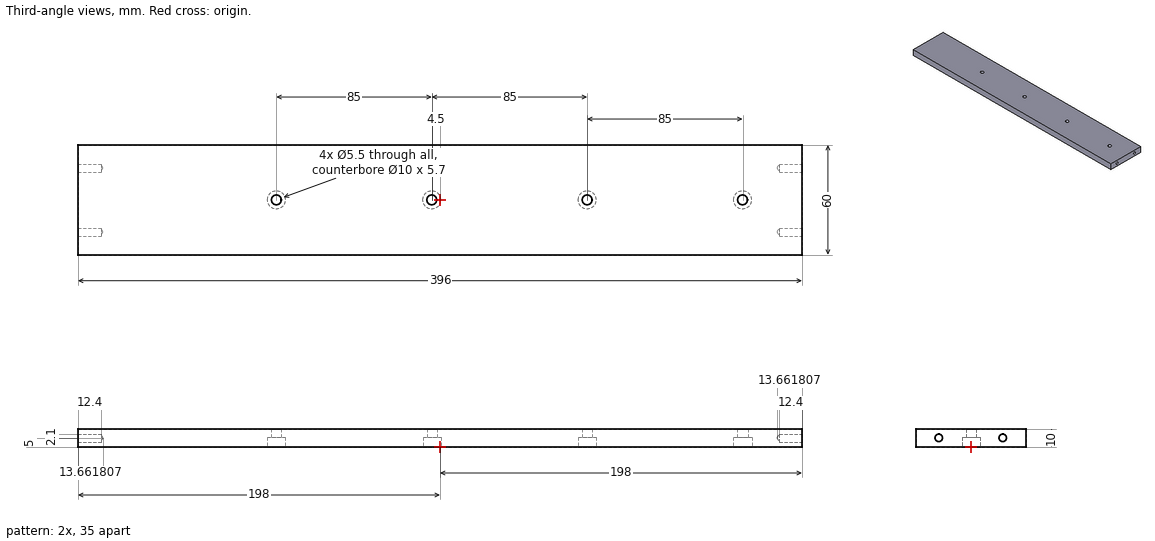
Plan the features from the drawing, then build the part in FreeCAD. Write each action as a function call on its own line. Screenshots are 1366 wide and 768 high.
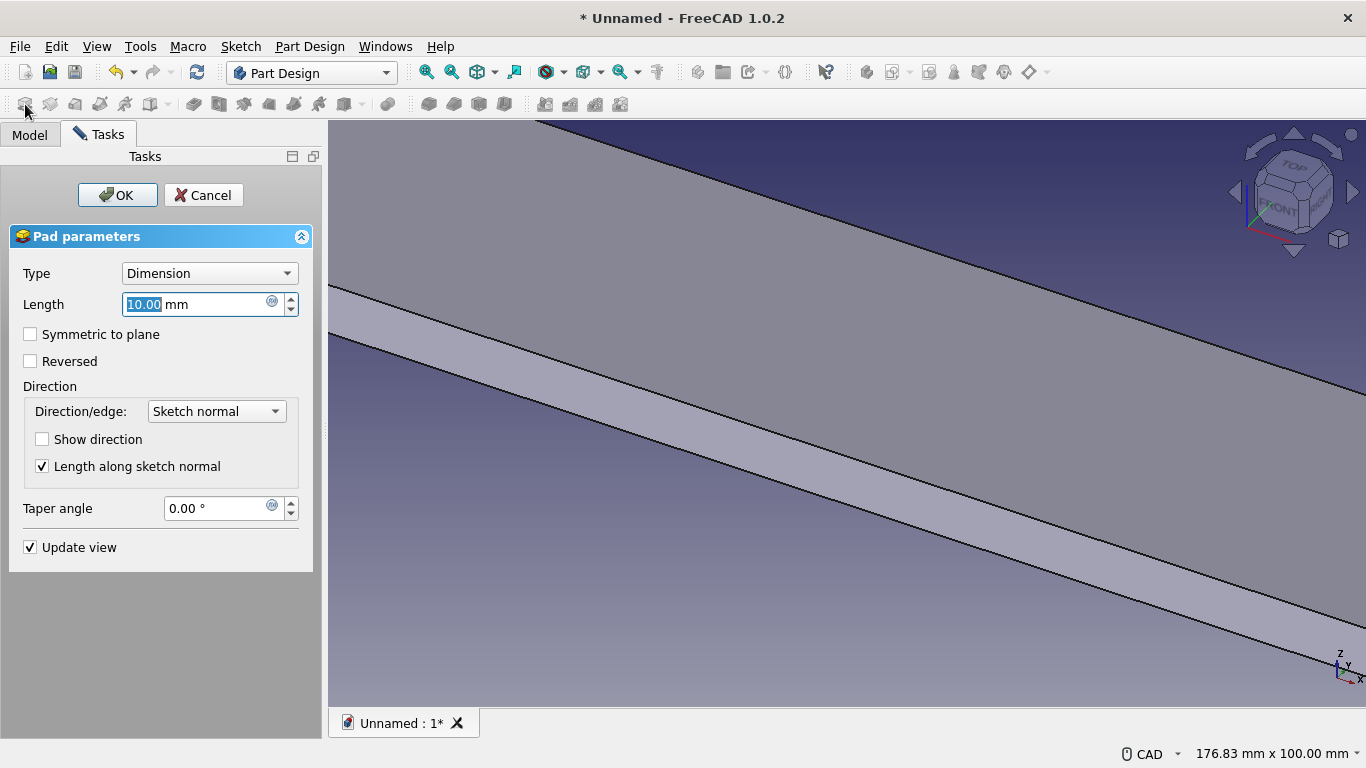
text(10)
key(Tab)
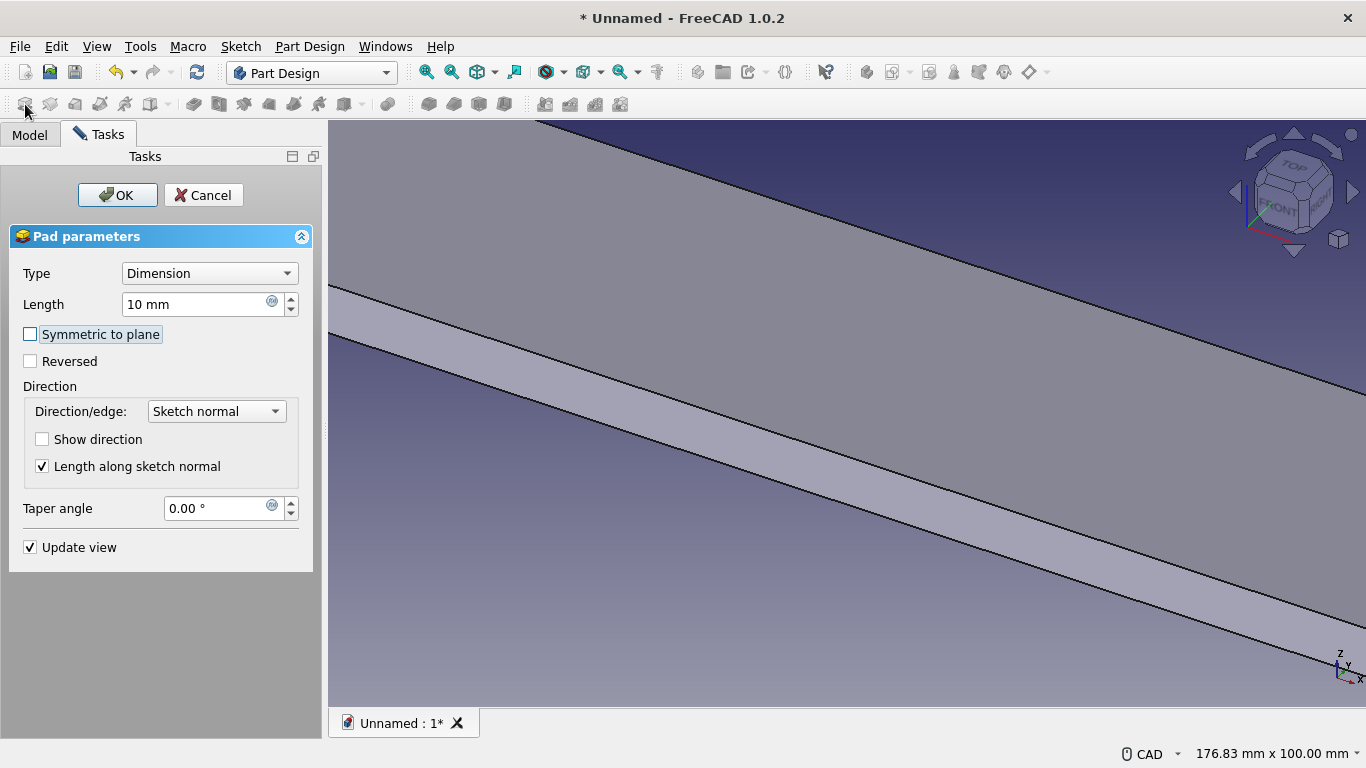
click(118, 195)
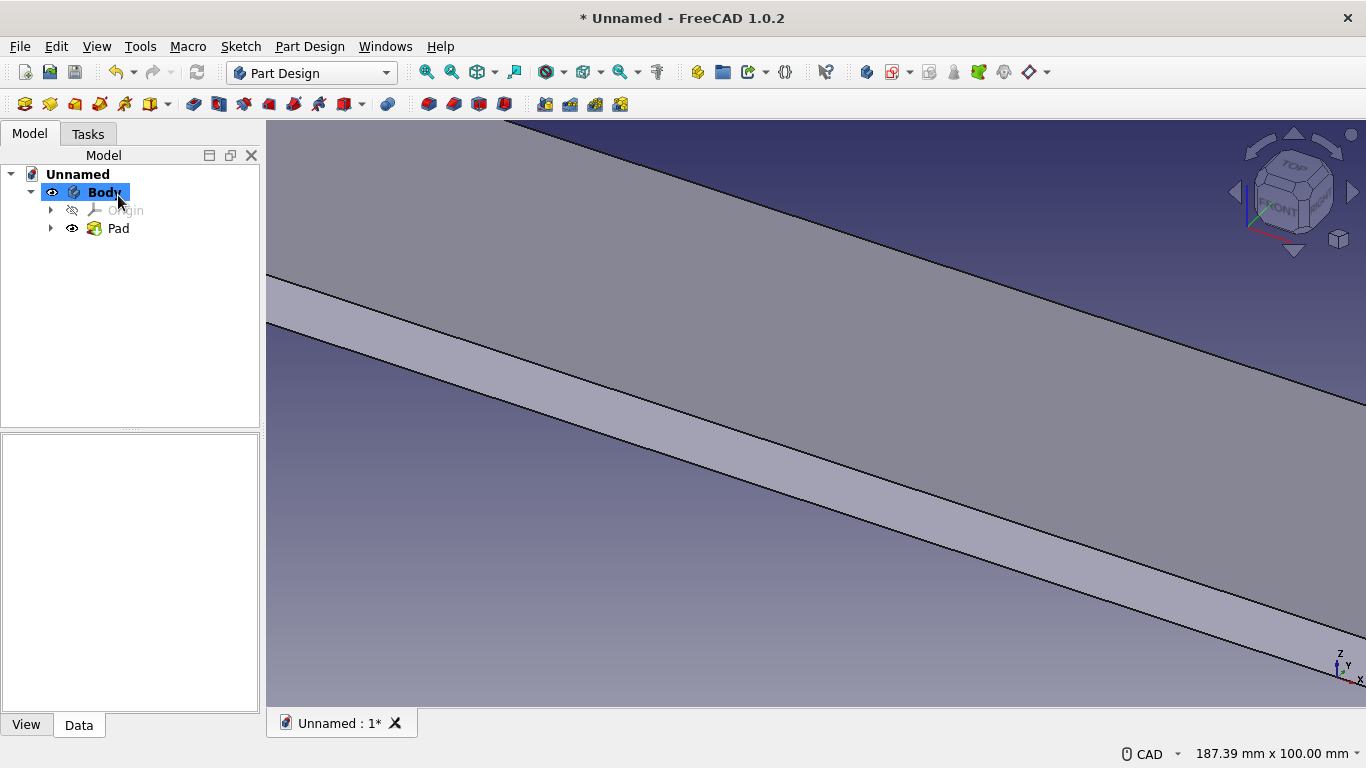
click(427, 72)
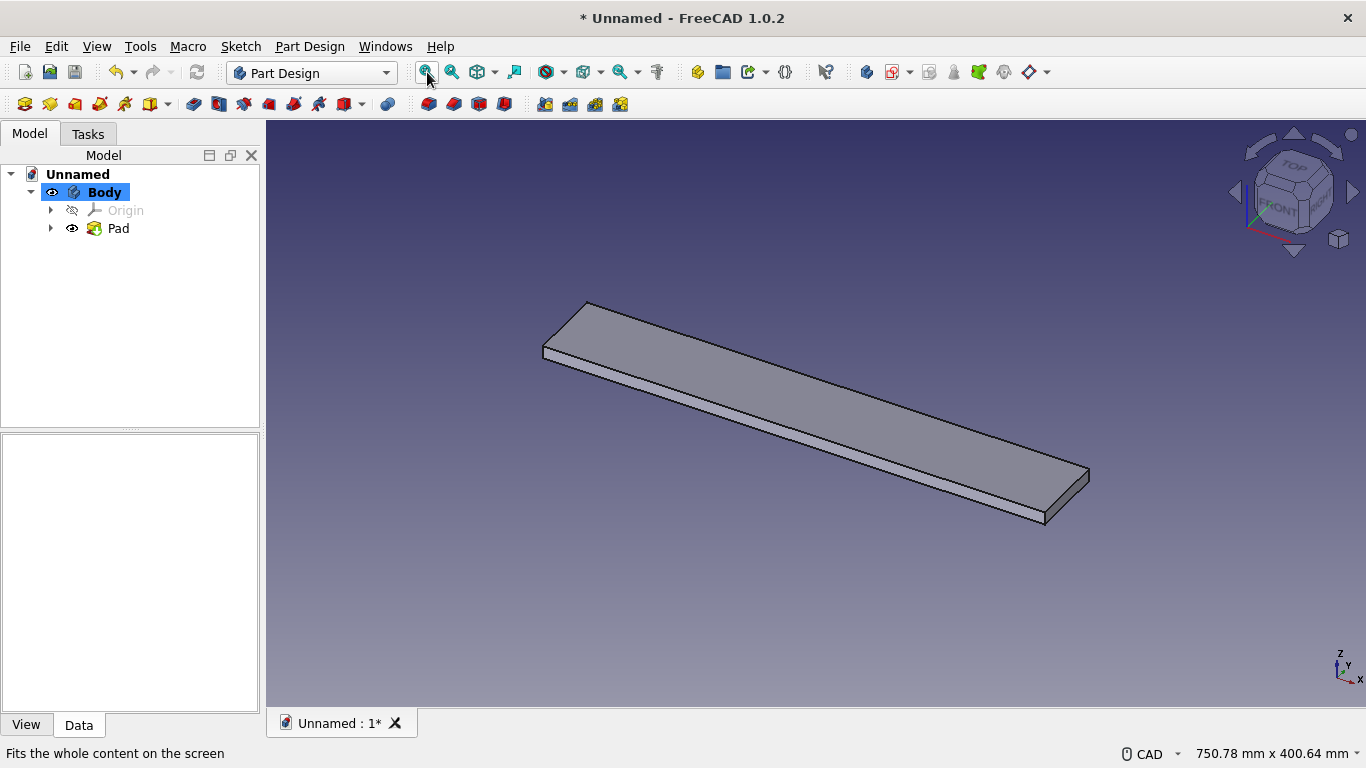
click(892, 72)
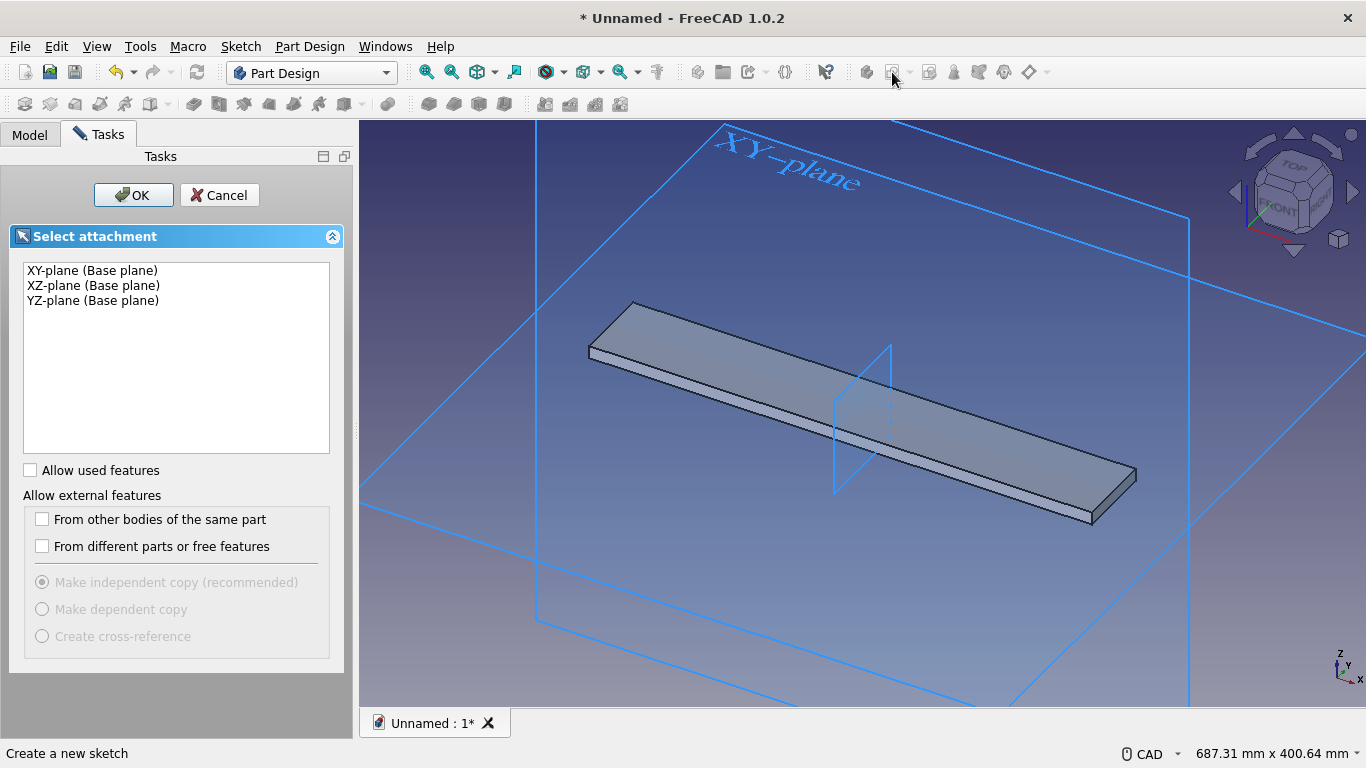
click(84, 270)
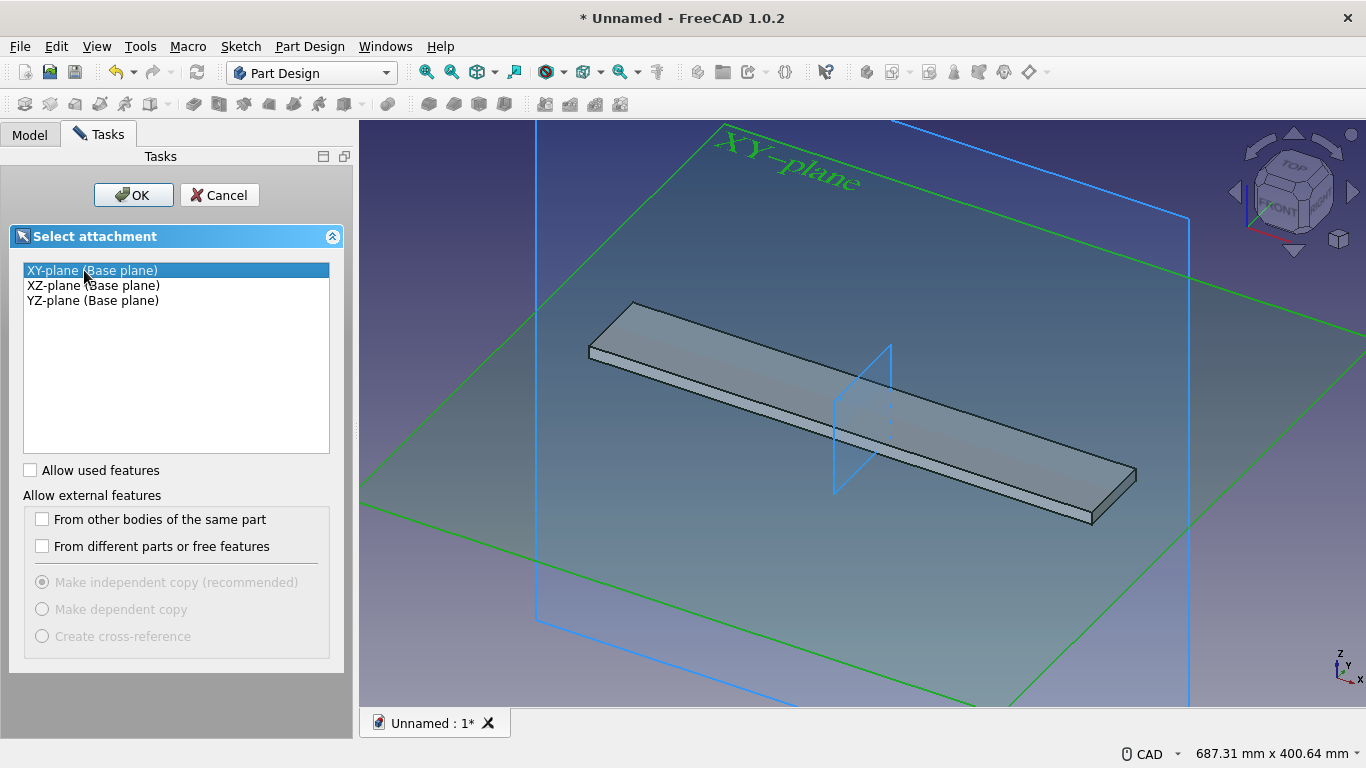
click(134, 195)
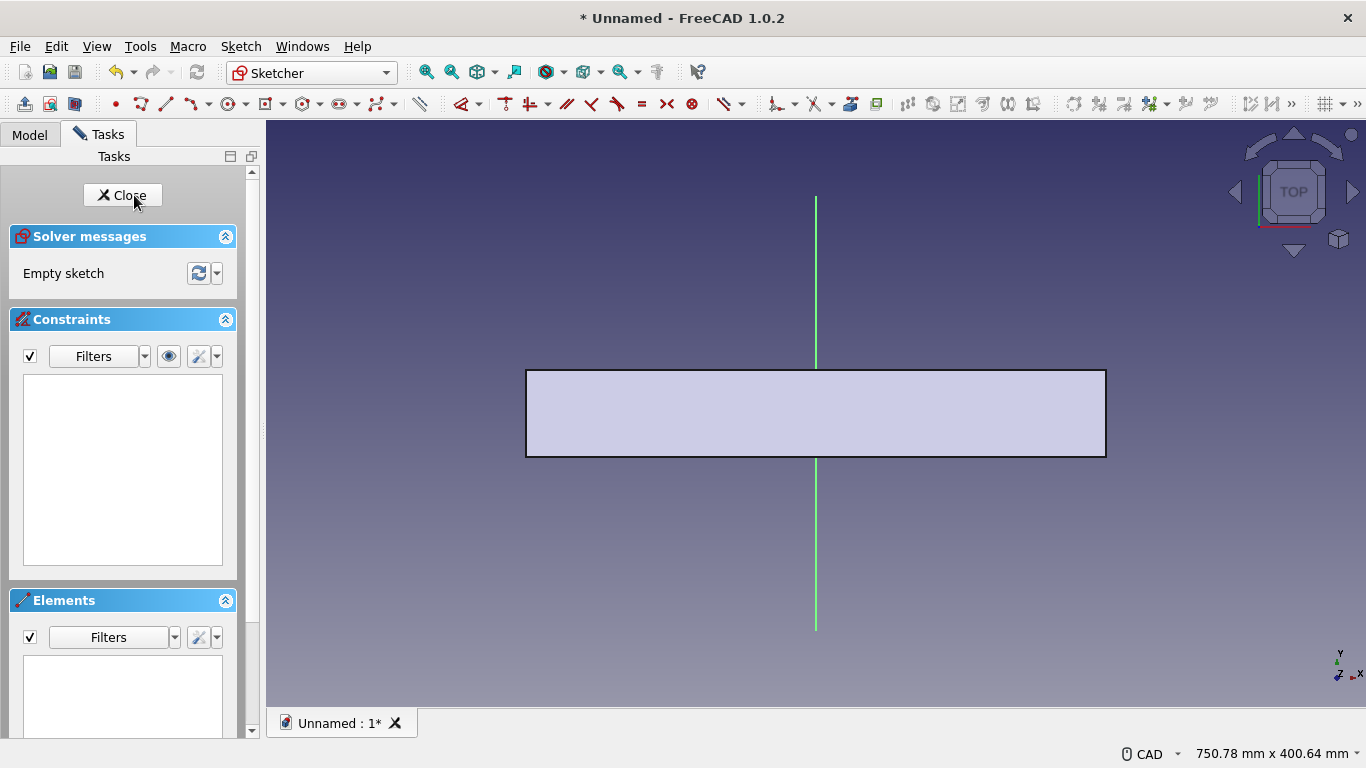
click(75, 104)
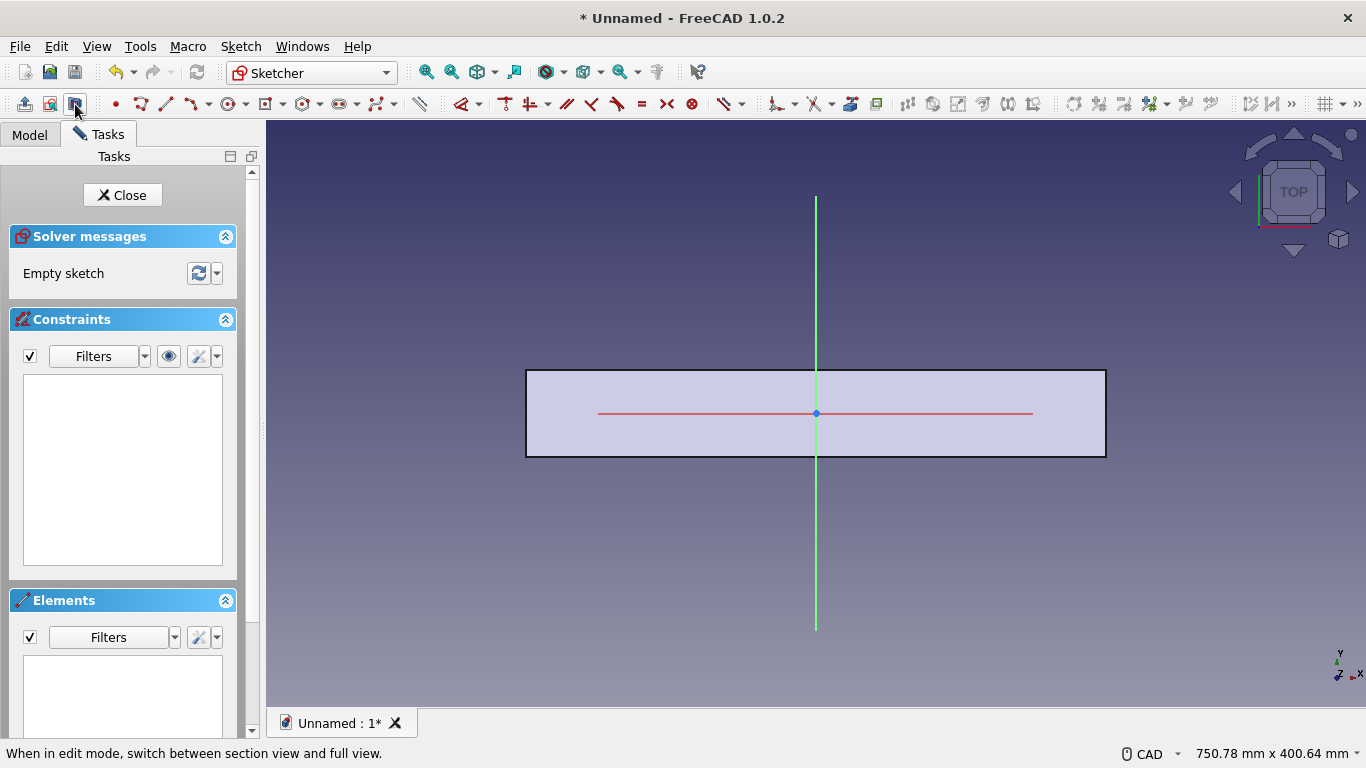
scroll(1023, 414, up, 3)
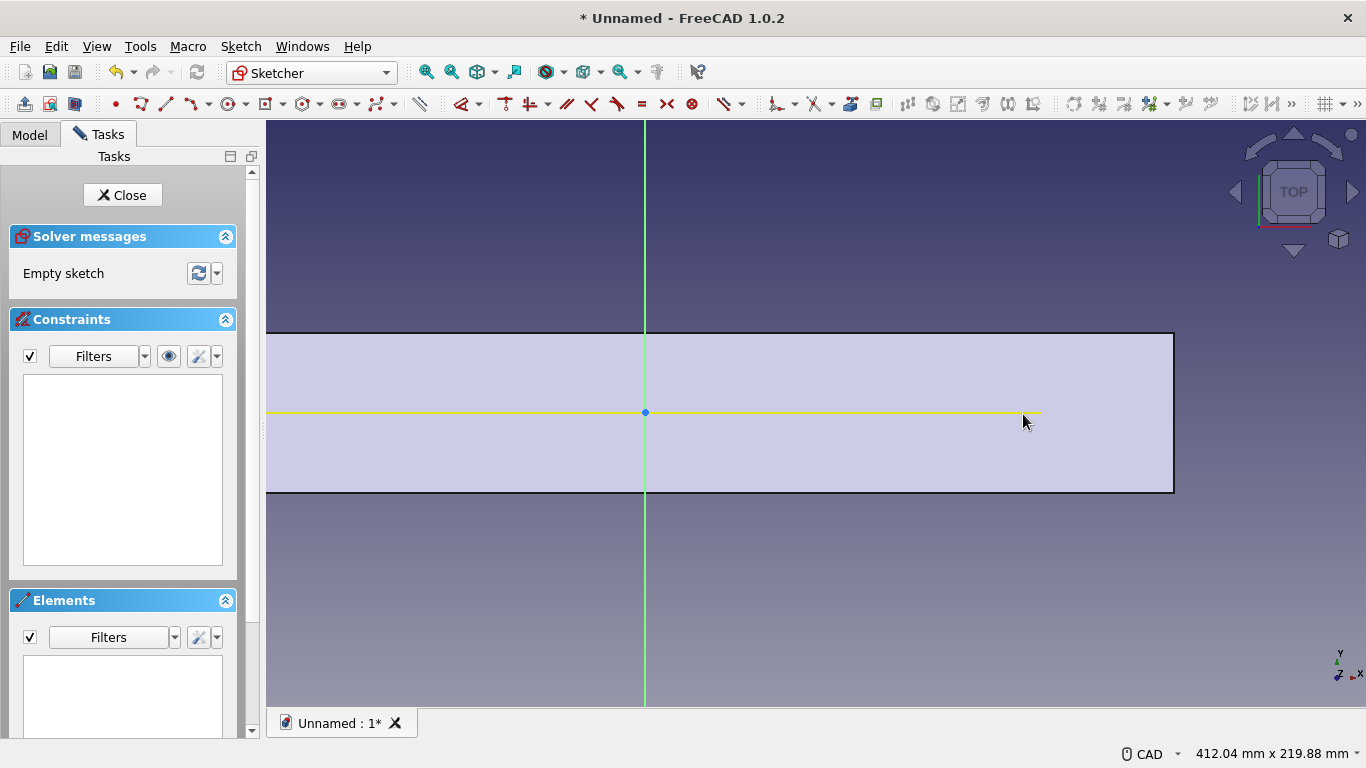
click(228, 104)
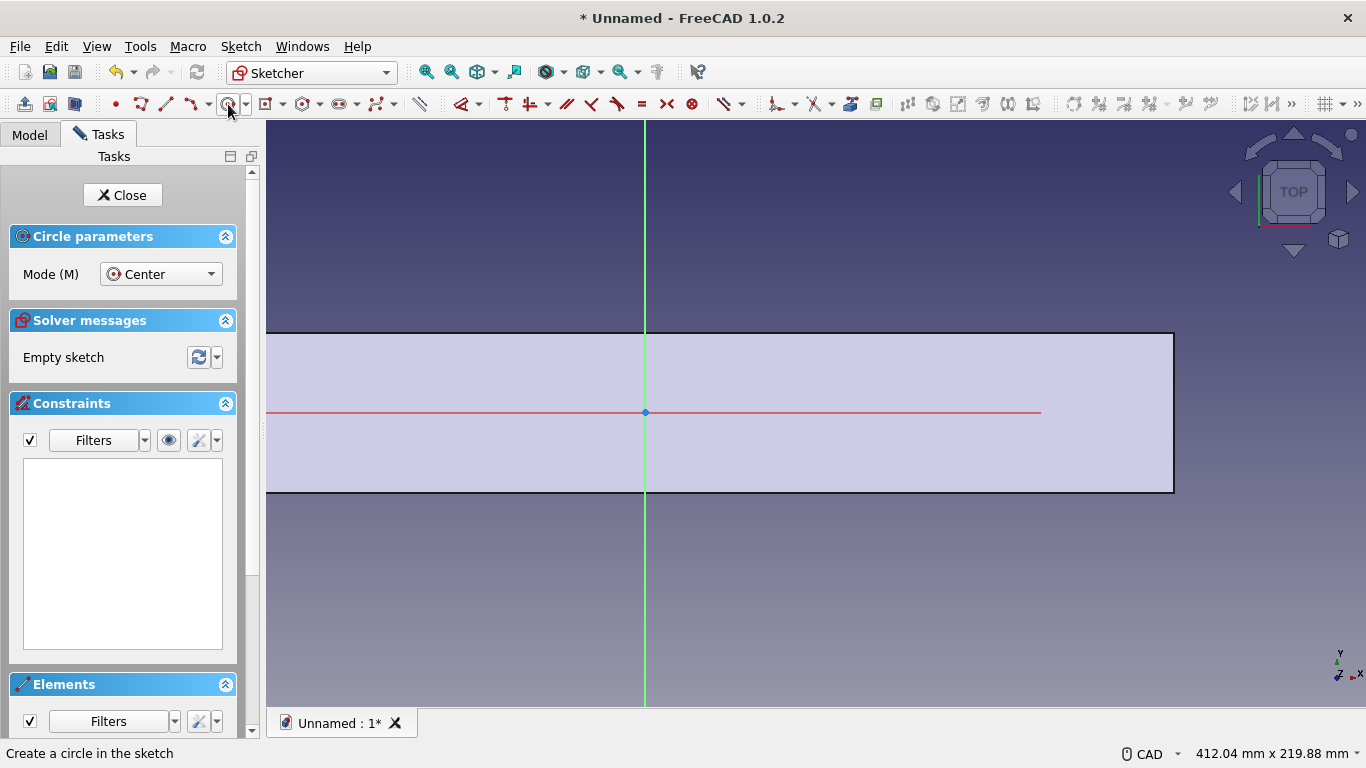
scroll(406, 413, up, 6)